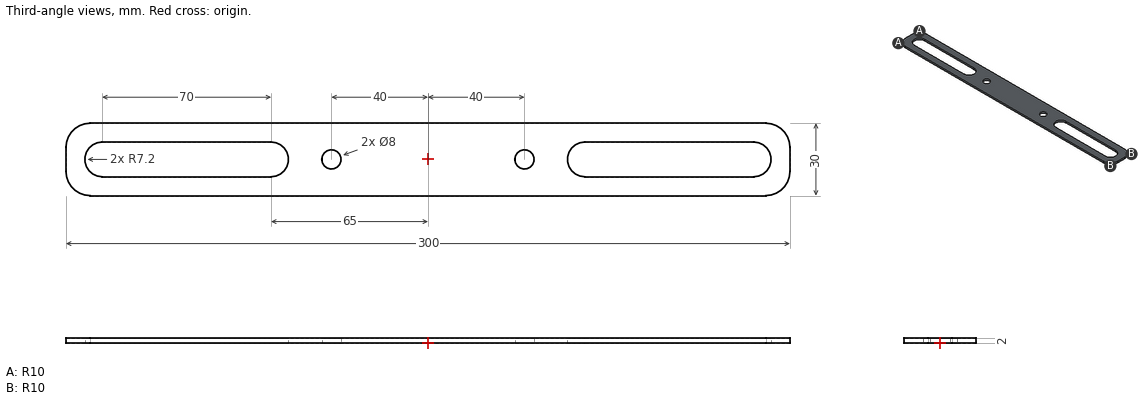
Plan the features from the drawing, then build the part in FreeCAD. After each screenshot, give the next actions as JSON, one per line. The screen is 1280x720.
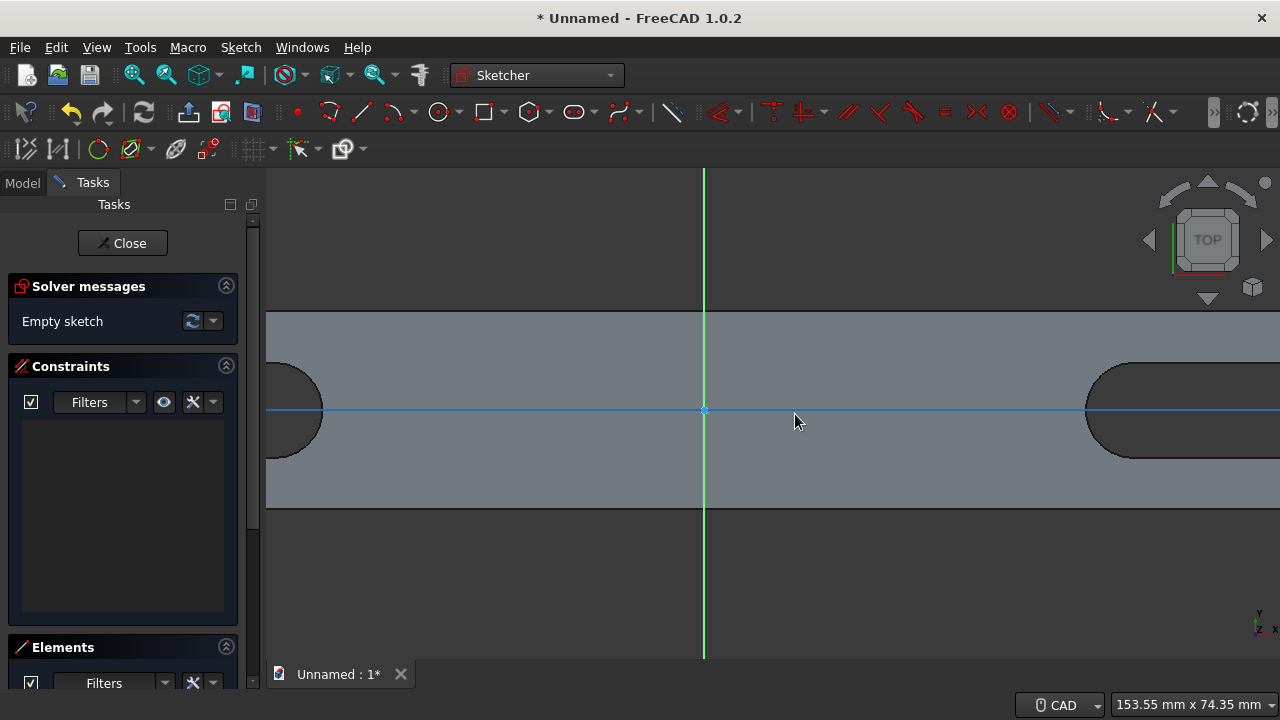
{"action": "left_click", "coordinate": [440, 112]}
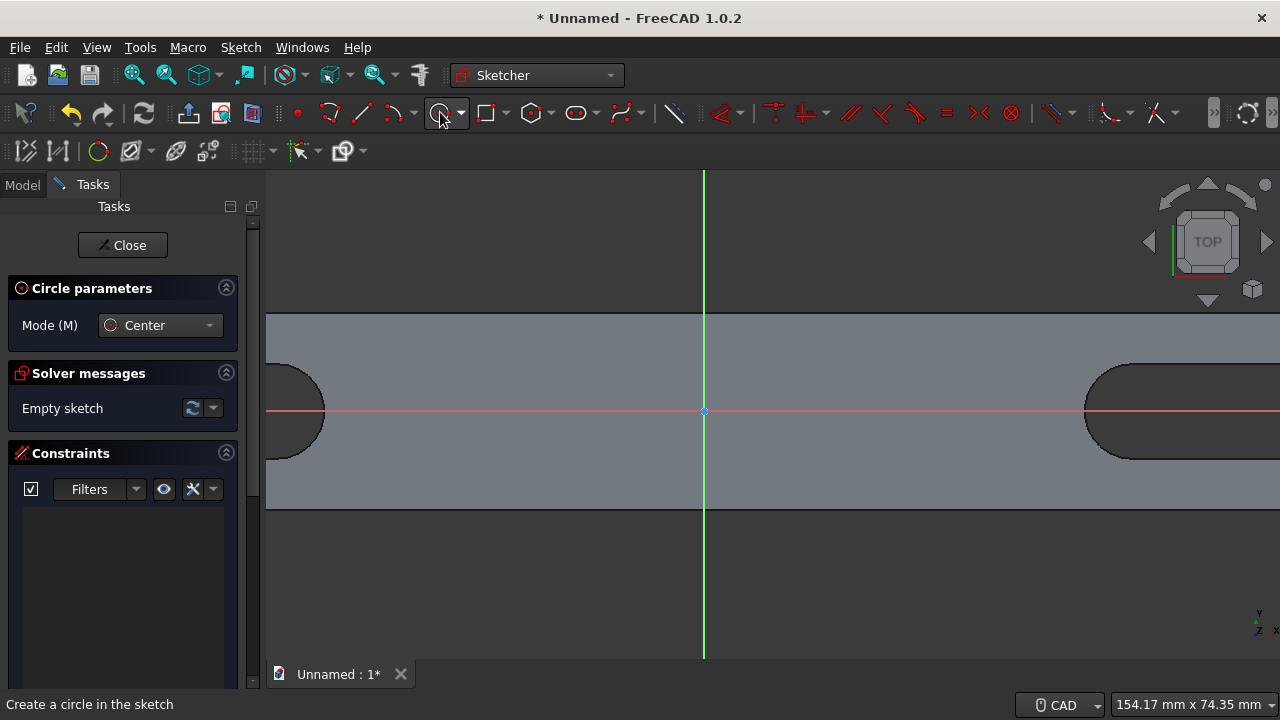
{"action": "left_click", "coordinate": [441, 411]}
{"action": "left_click", "coordinate": [460, 393]}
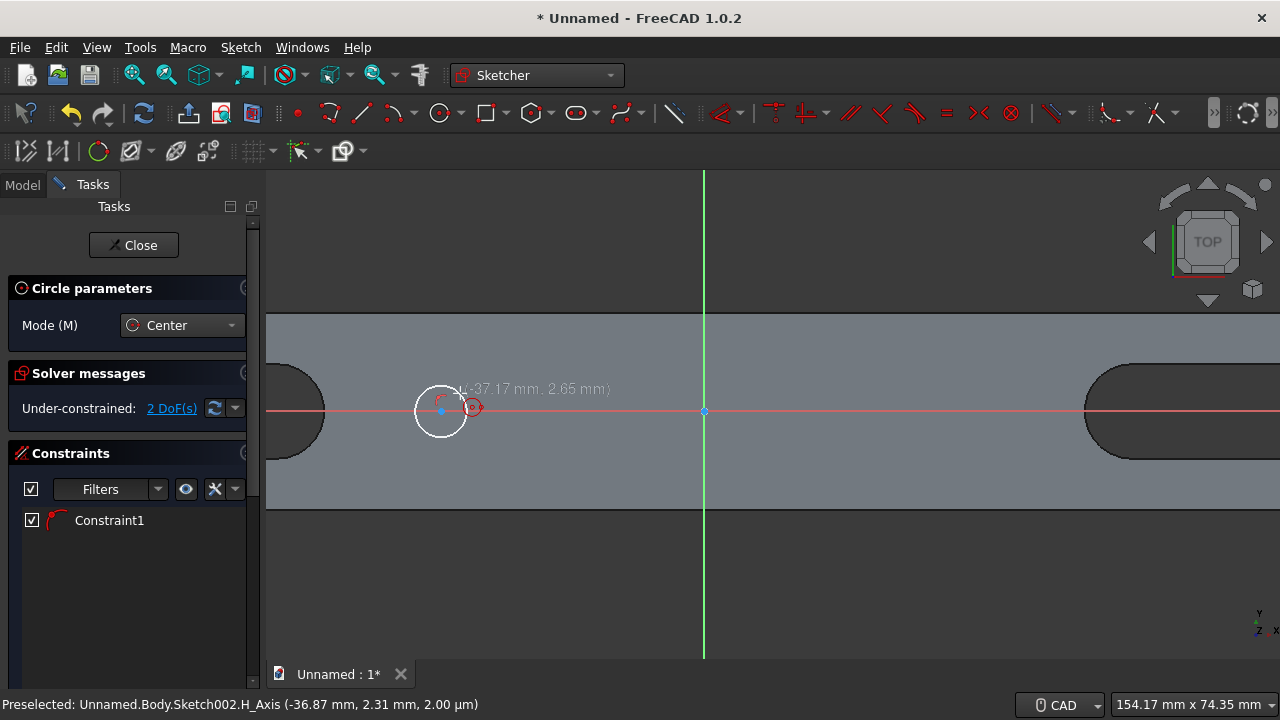
{"action": "left_click", "coordinate": [968, 411]}
{"action": "left_click", "coordinate": [986, 393]}
{"action": "key", "text": "Escape"}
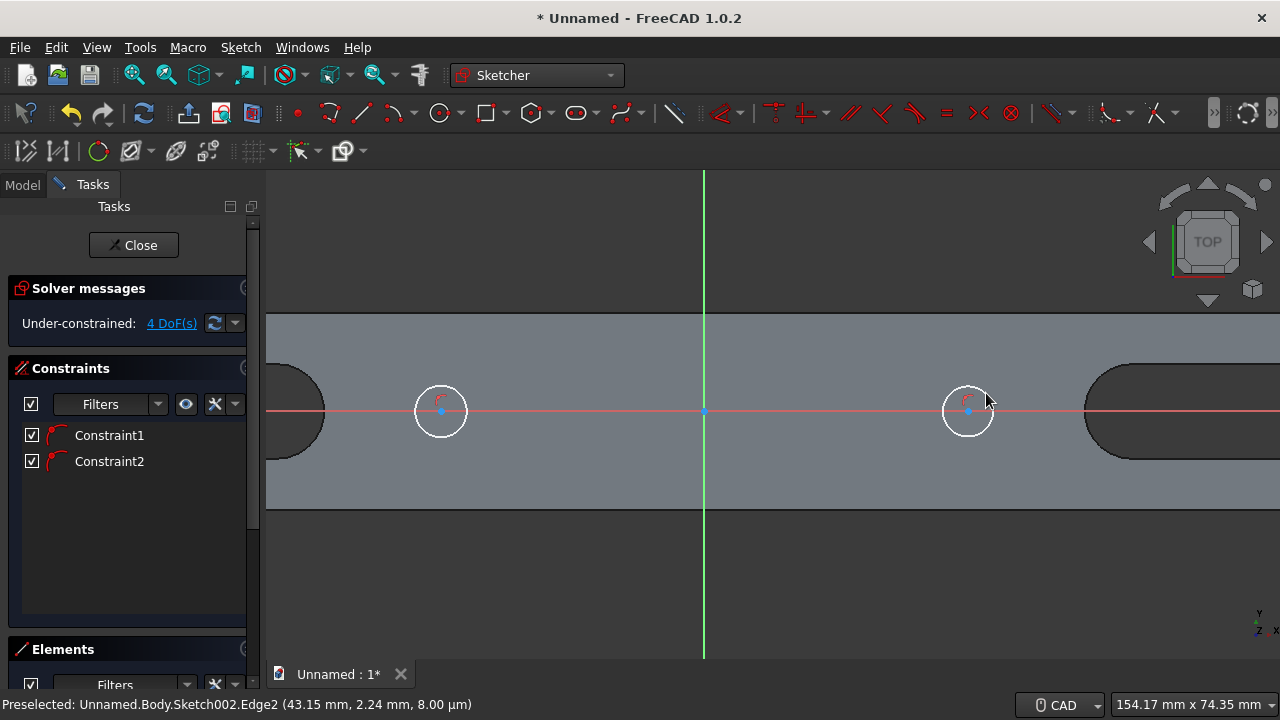
{"action": "left_click", "coordinate": [459, 393]}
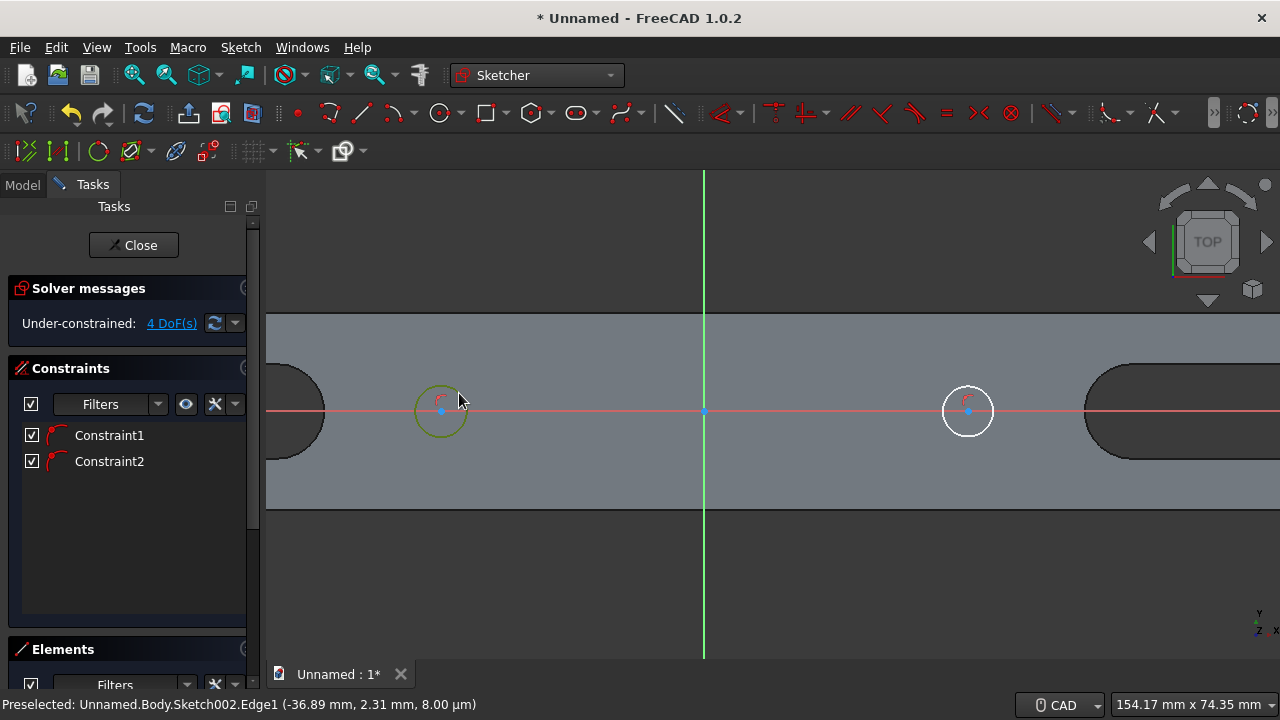
{"action": "left_click", "coordinate": [986, 394]}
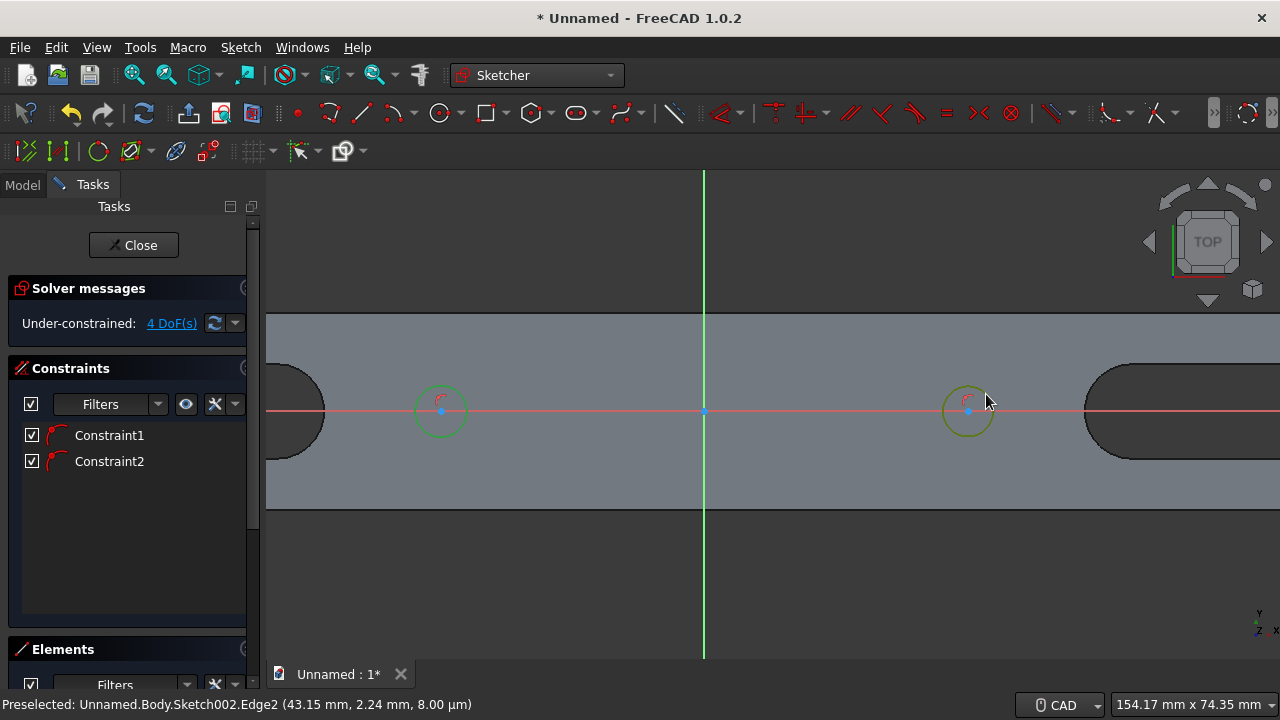
{"action": "key", "text": "e"}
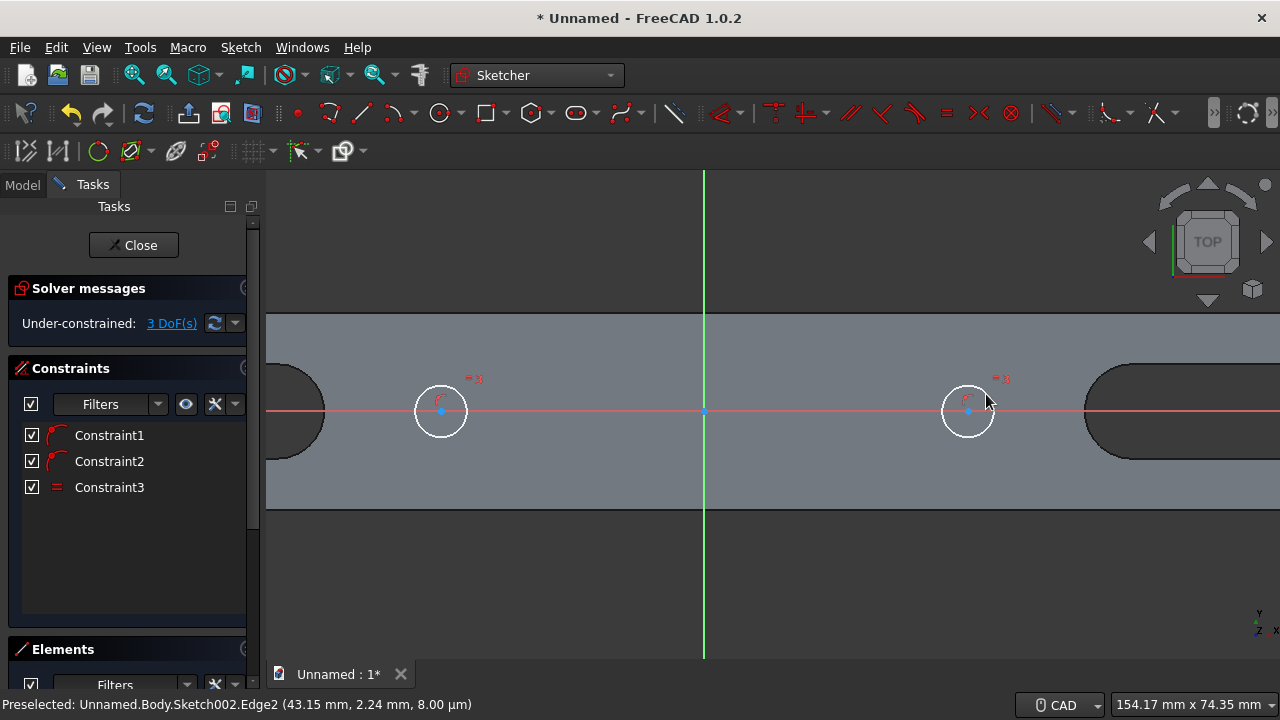
{"action": "left_click", "coordinate": [459, 393]}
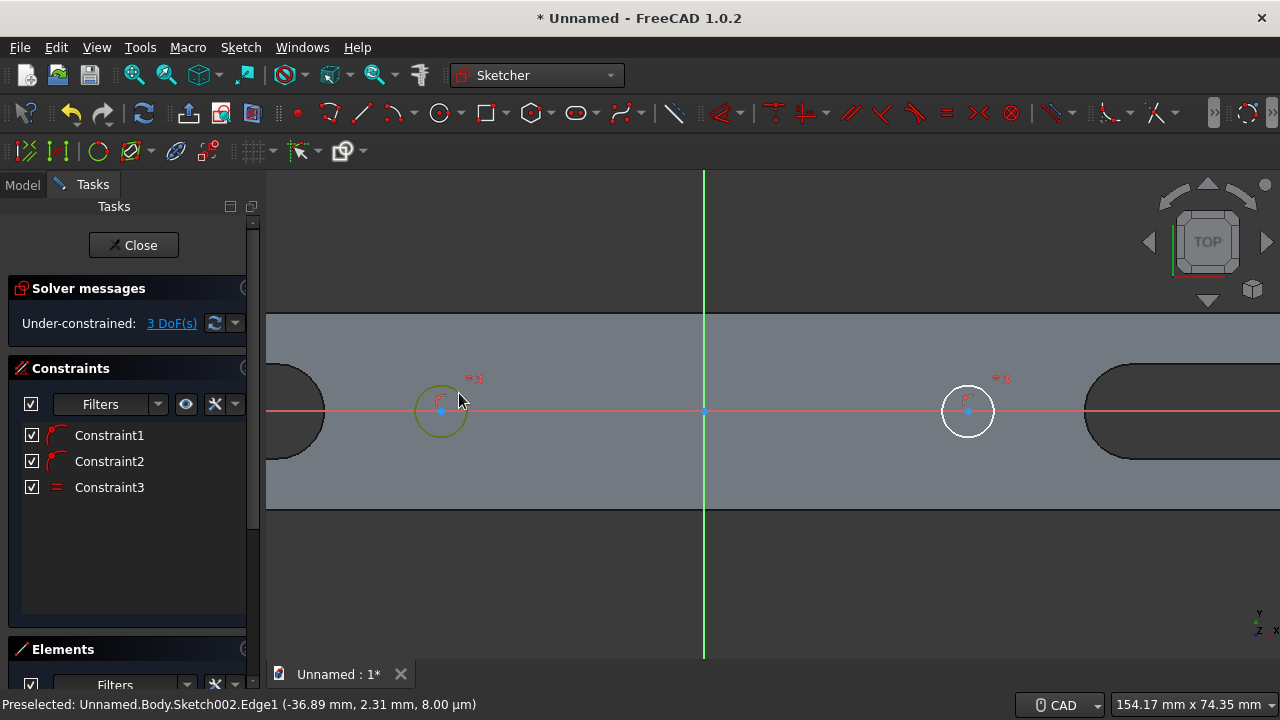
{"action": "key", "text": "k o"}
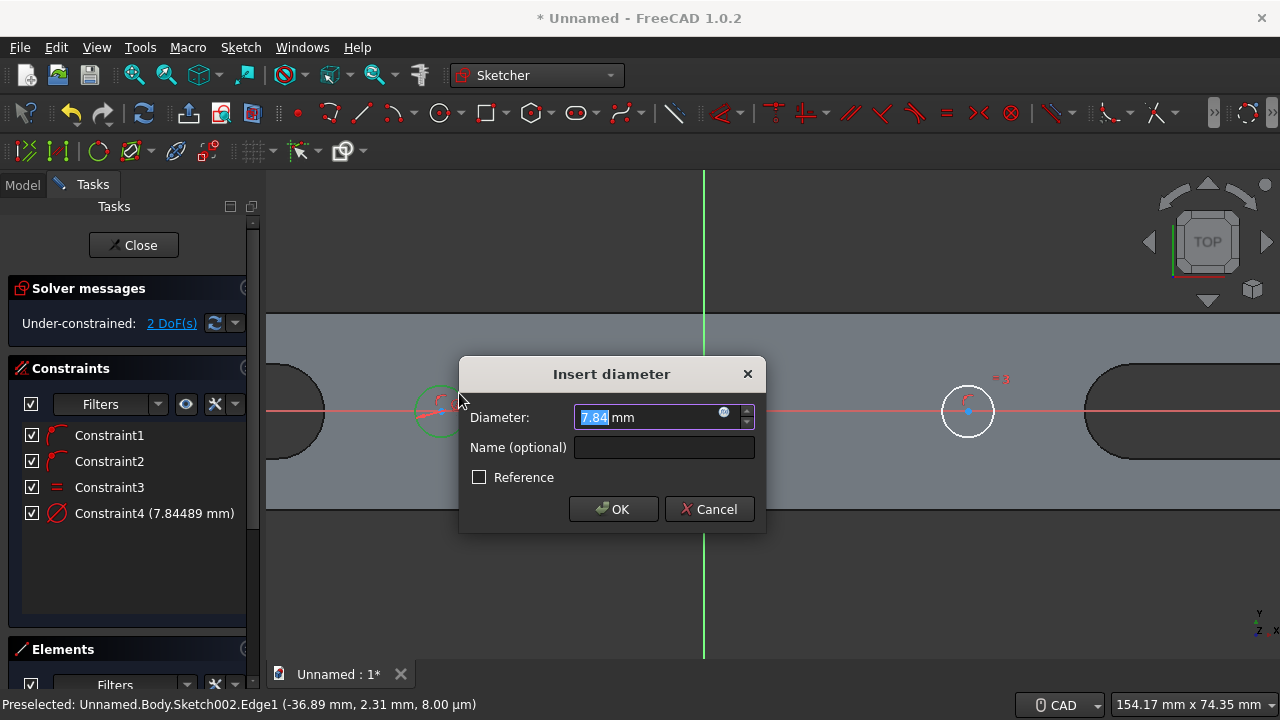
{"action": "type", "text": "8"}
{"action": "key", "text": "Return"}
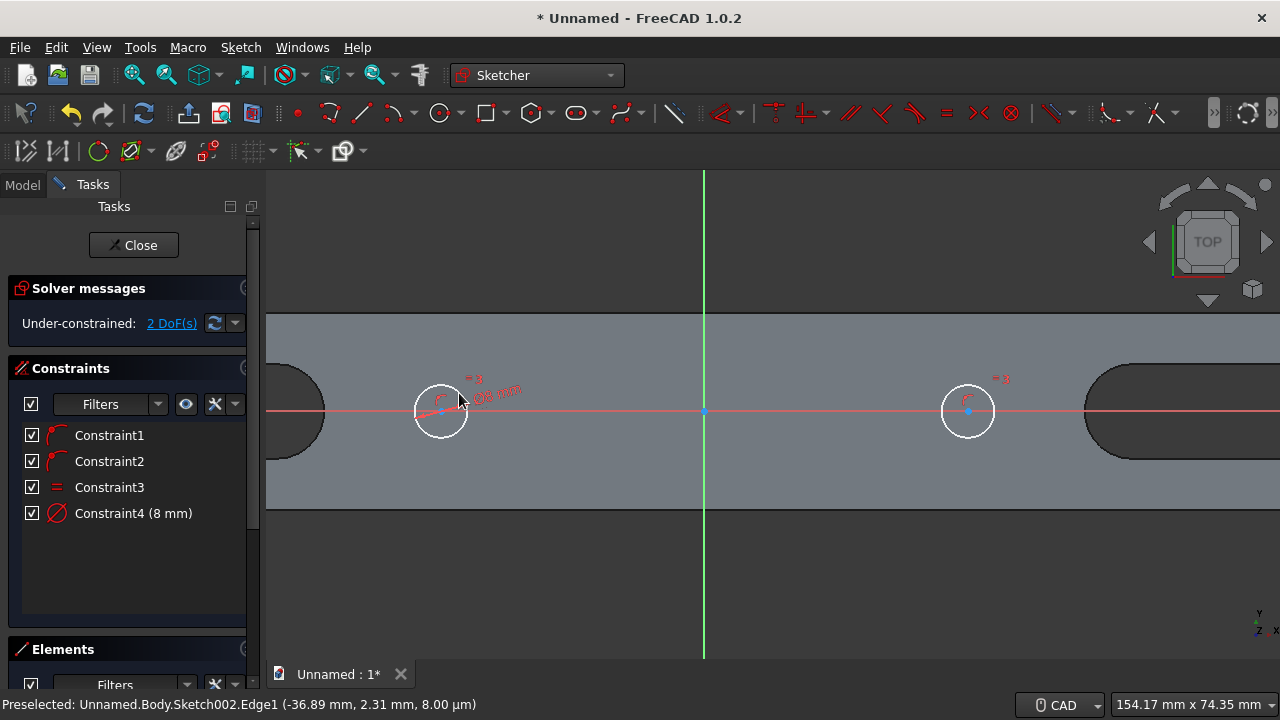
{"action": "left_click", "coordinate": [441, 411]}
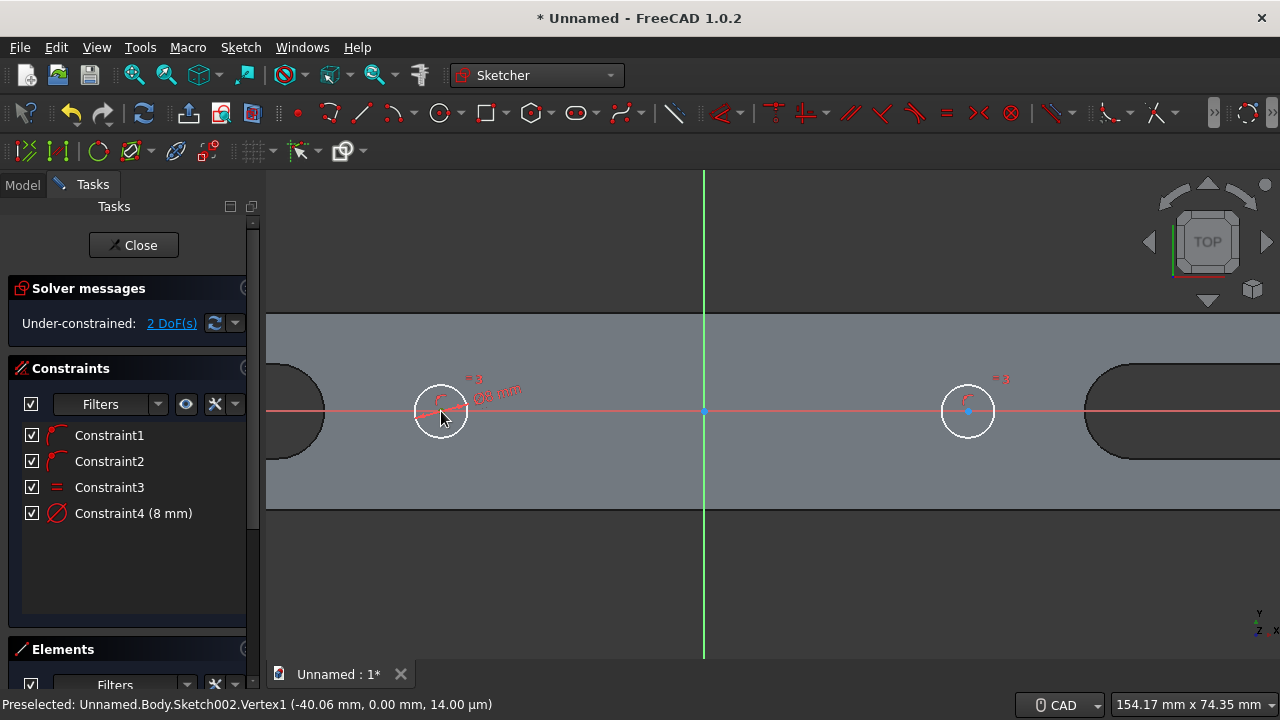
{"action": "key", "text": "l"}